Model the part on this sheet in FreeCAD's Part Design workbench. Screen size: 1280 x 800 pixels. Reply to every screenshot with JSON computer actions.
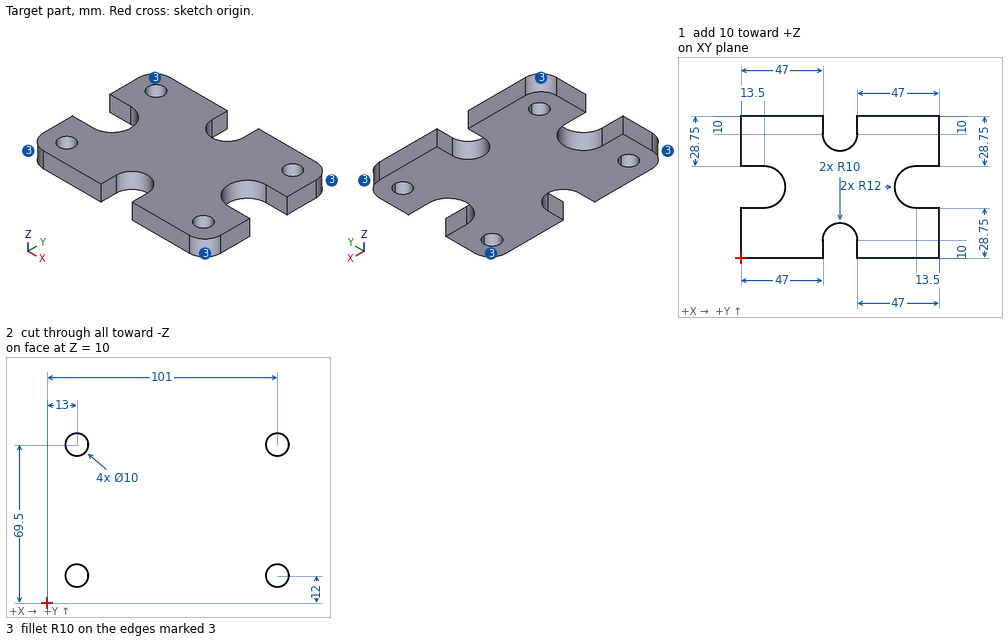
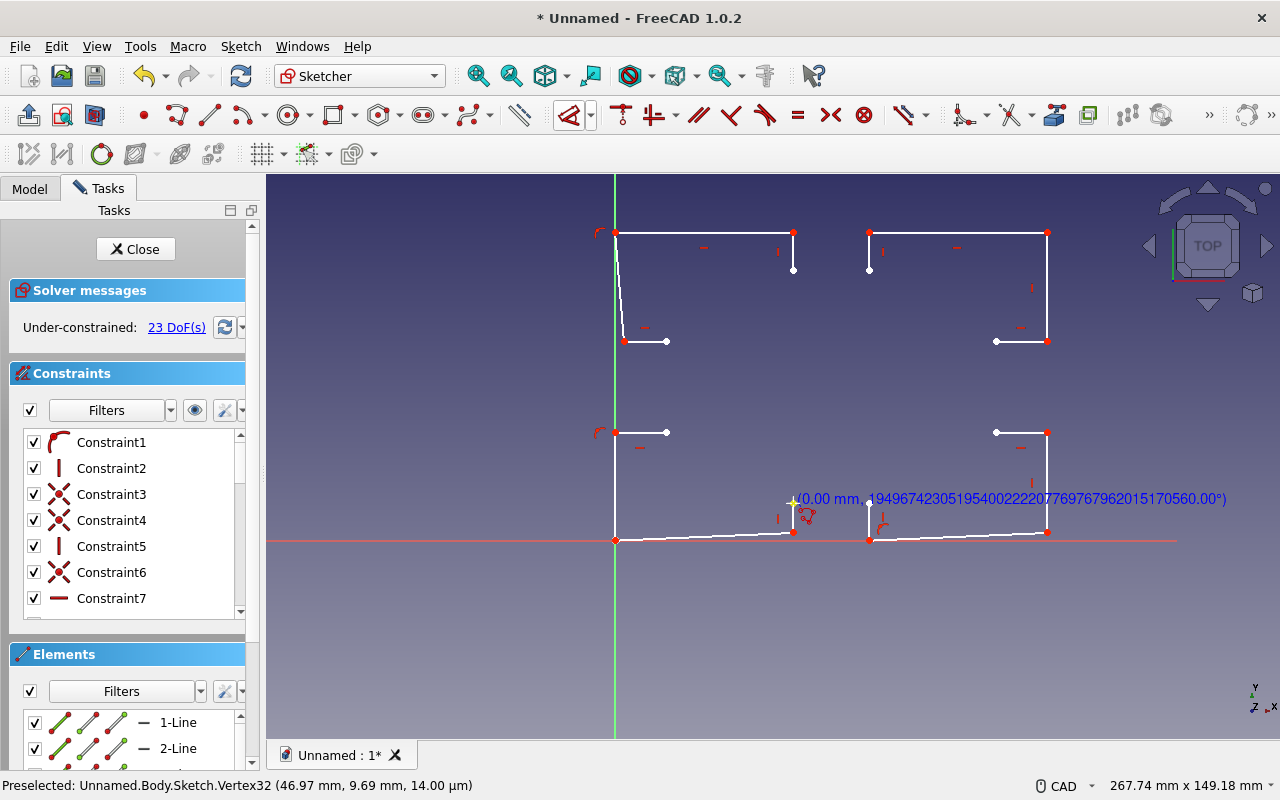
{"action": "left_click", "coordinate": [264, 116]}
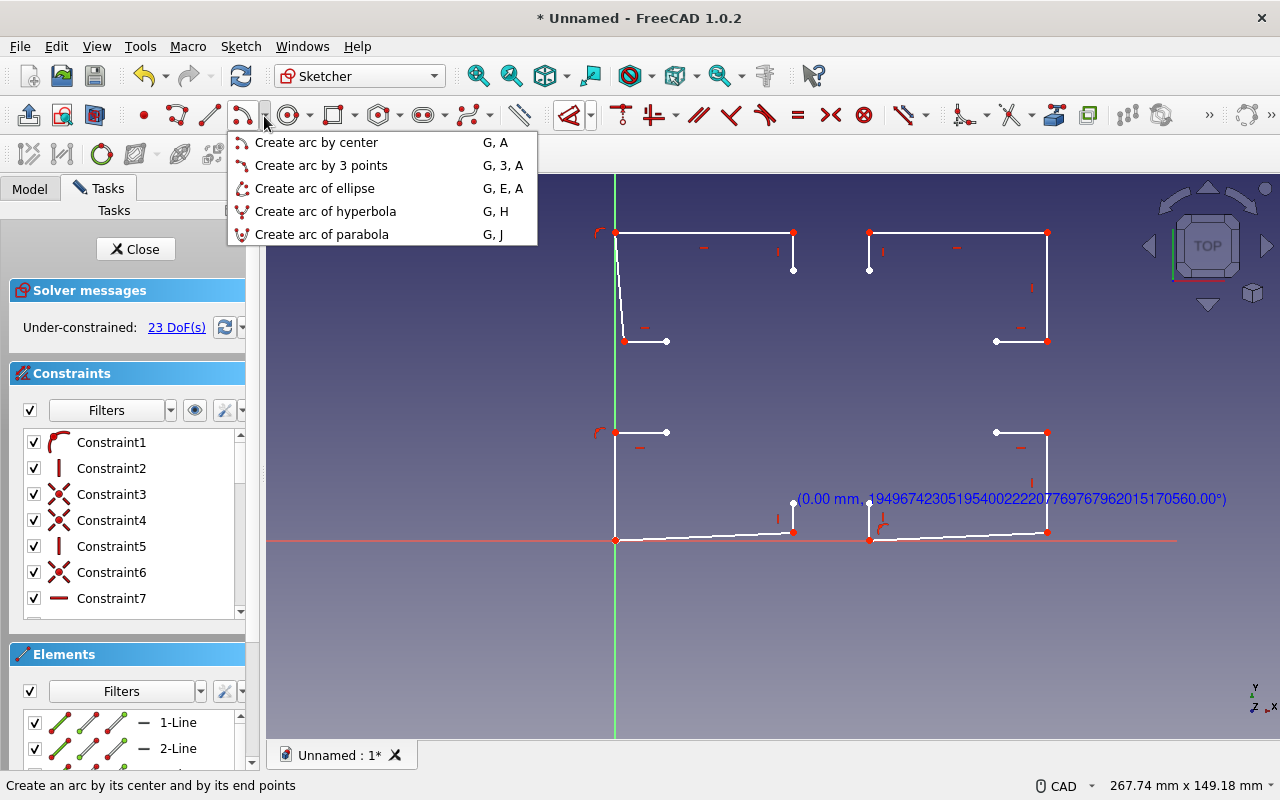
{"action": "left_click", "coordinate": [382, 166]}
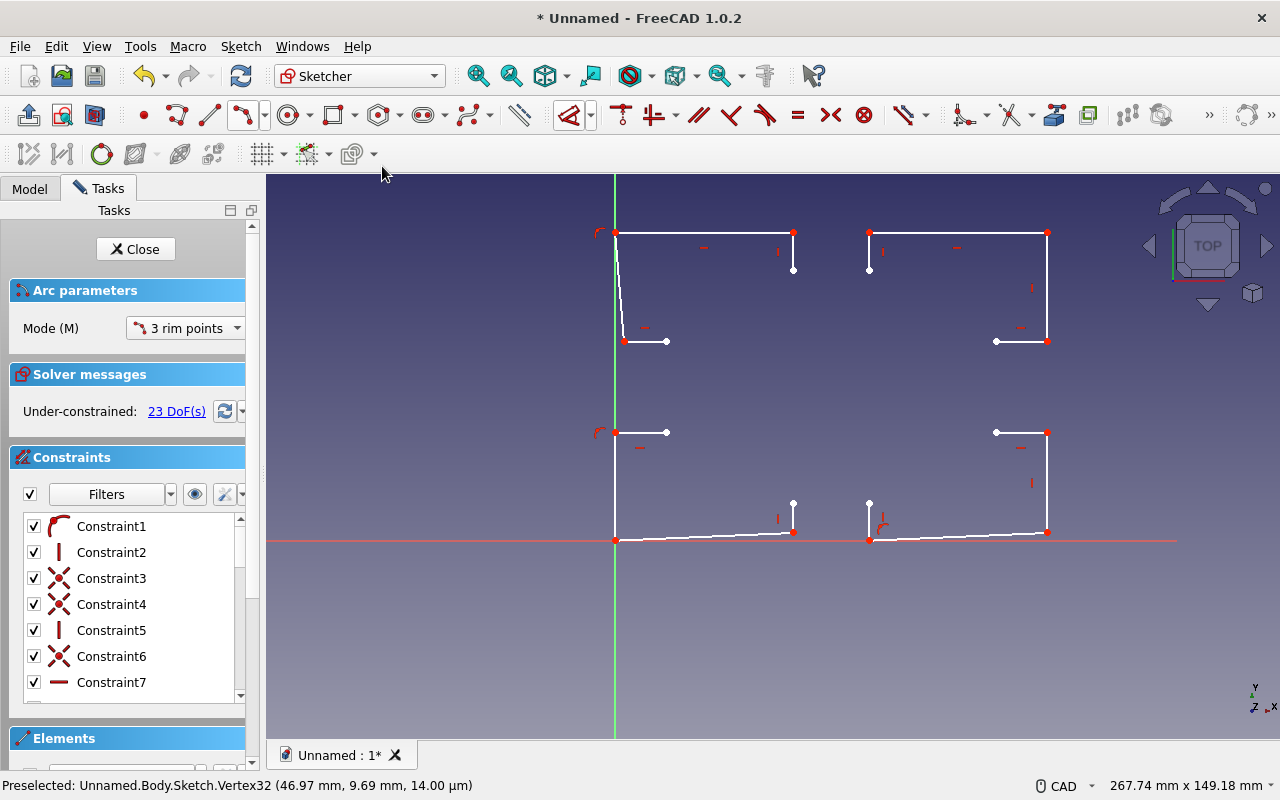
{"action": "left_click", "coordinate": [996, 433]}
{"action": "left_click", "coordinate": [996, 342]}
{"action": "left_click", "coordinate": [950, 386]}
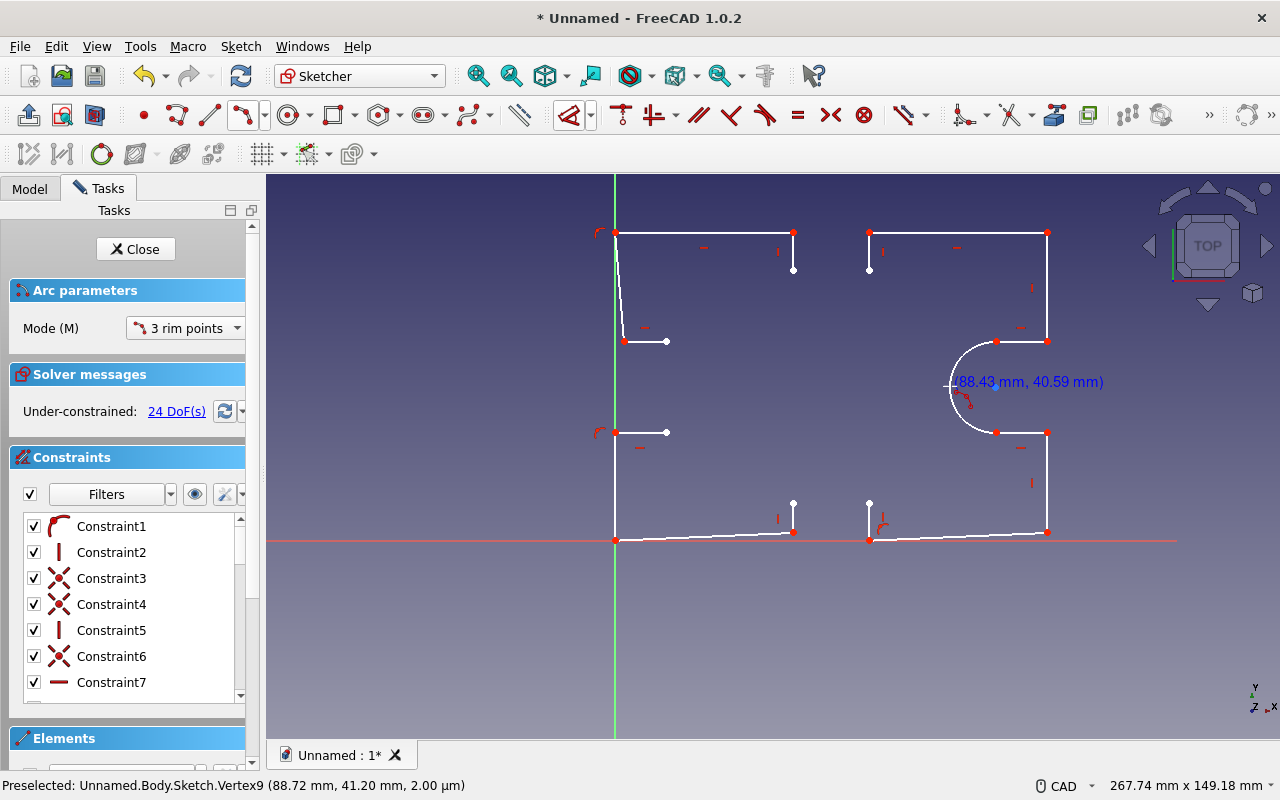
{"action": "left_click", "coordinate": [869, 271]}
{"action": "left_click", "coordinate": [793, 271]}
{"action": "left_click", "coordinate": [831, 308]}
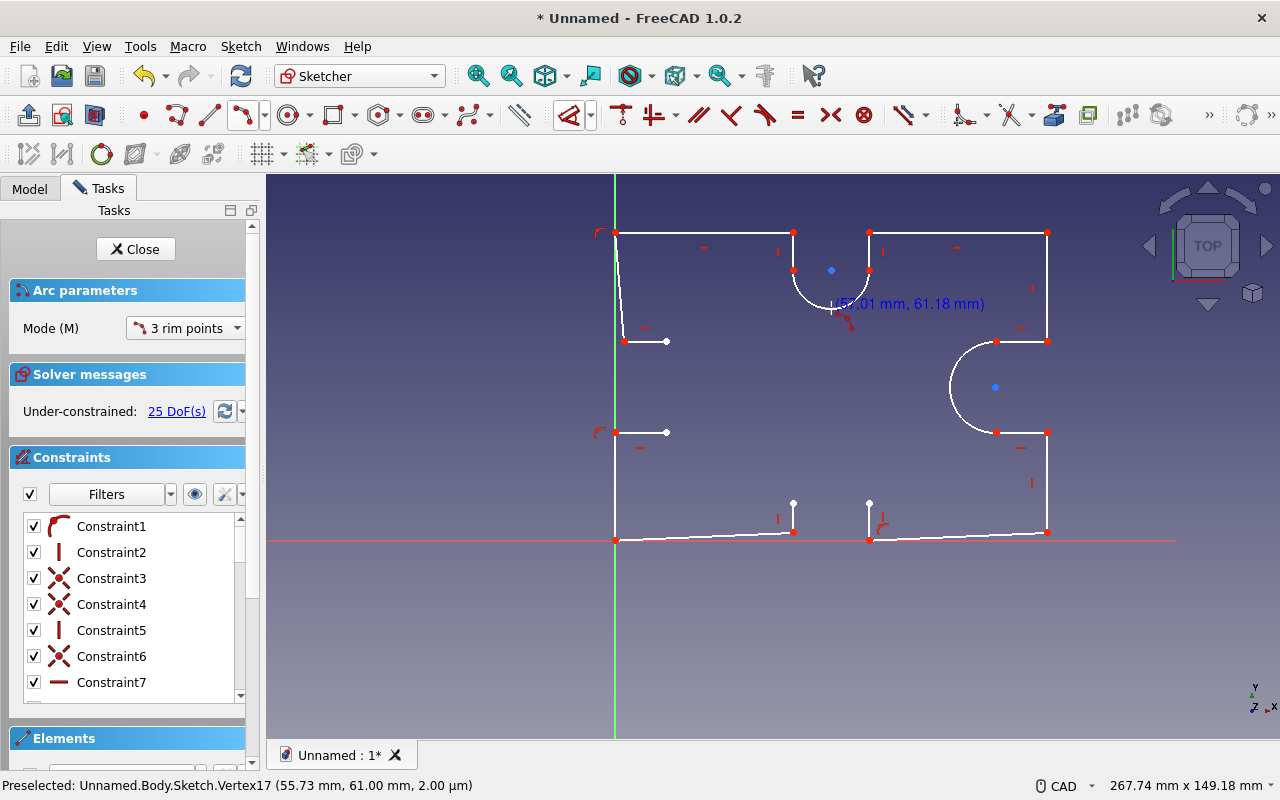
{"action": "left_click", "coordinate": [666, 342]}
{"action": "left_click", "coordinate": [666, 433]}
{"action": "left_click", "coordinate": [712, 386]}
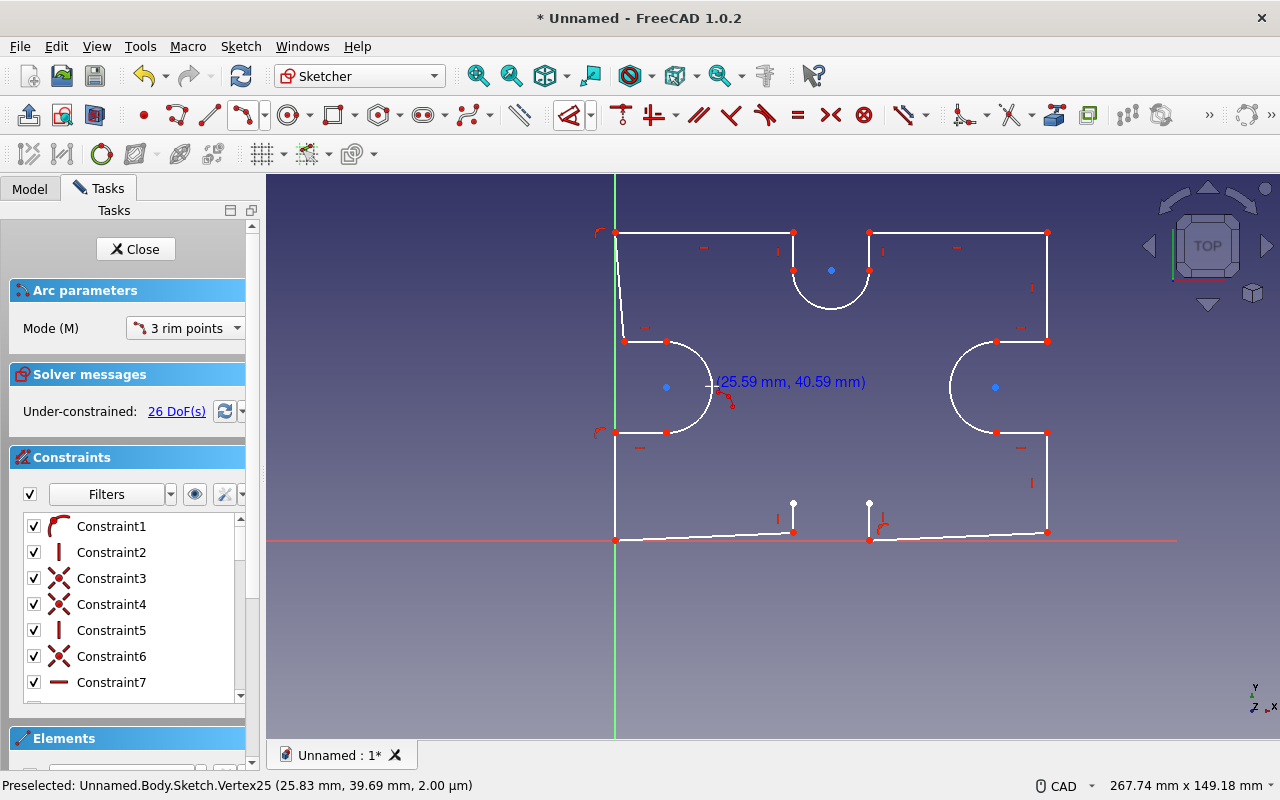
{"action": "left_click", "coordinate": [793, 504]}
{"action": "left_click", "coordinate": [869, 504]}
{"action": "left_click", "coordinate": [831, 465]}
{"action": "key", "text": "Escape"}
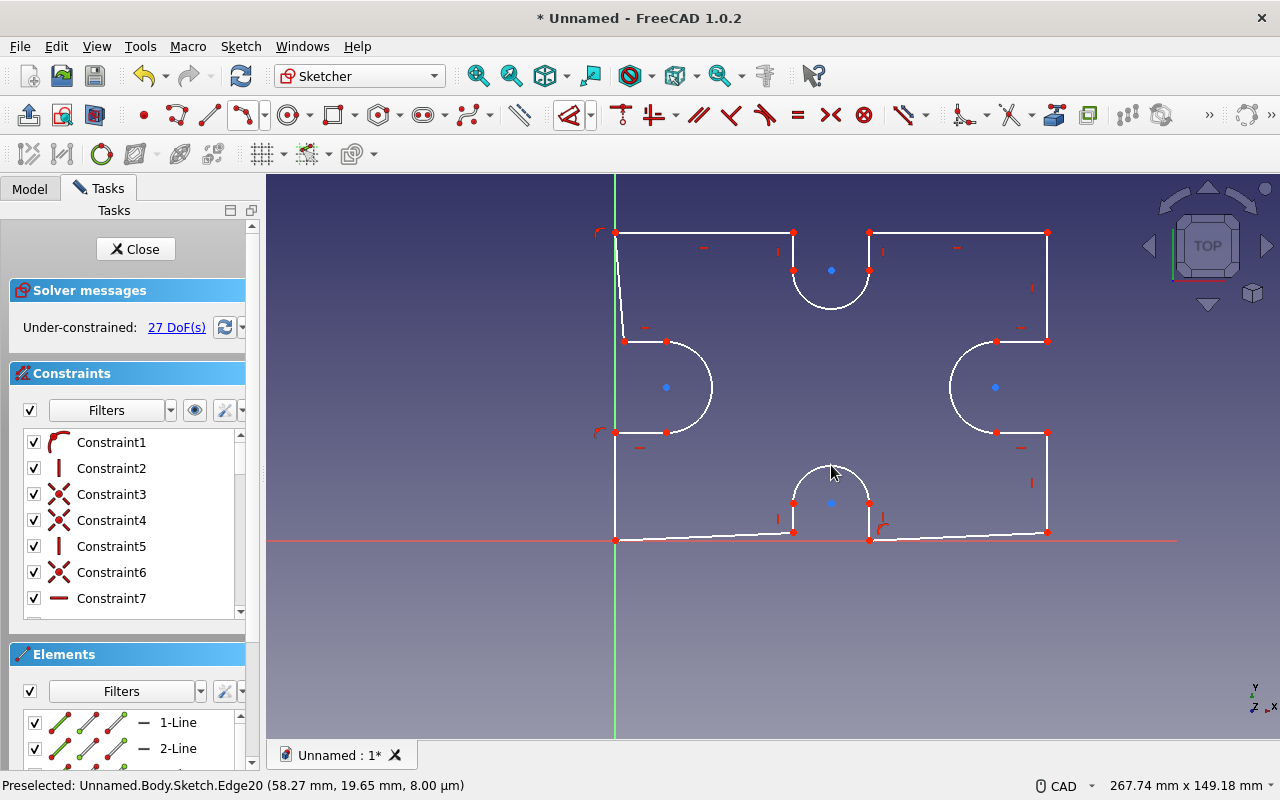
{"action": "scroll", "coordinate": [869, 515], "scroll_direction": "up", "scroll_amount": 2}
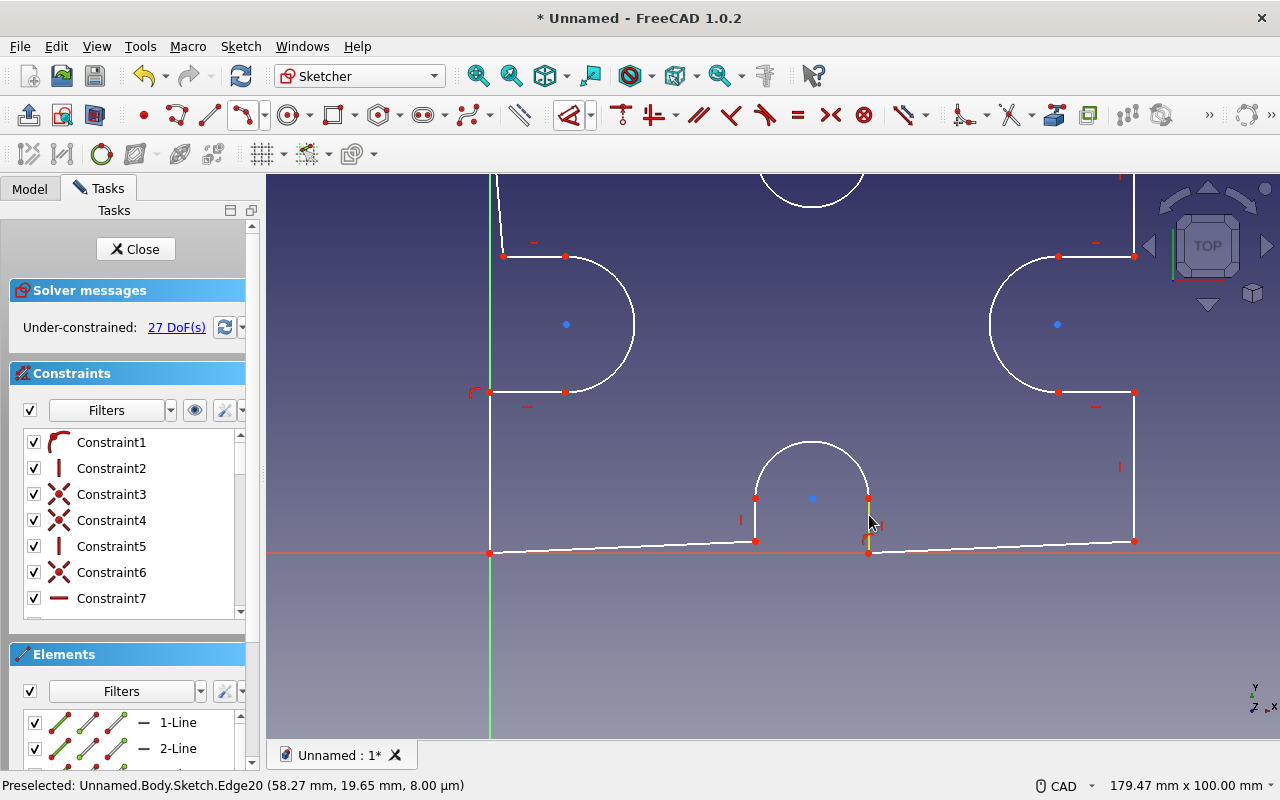
{"action": "left_click", "coordinate": [869, 515]}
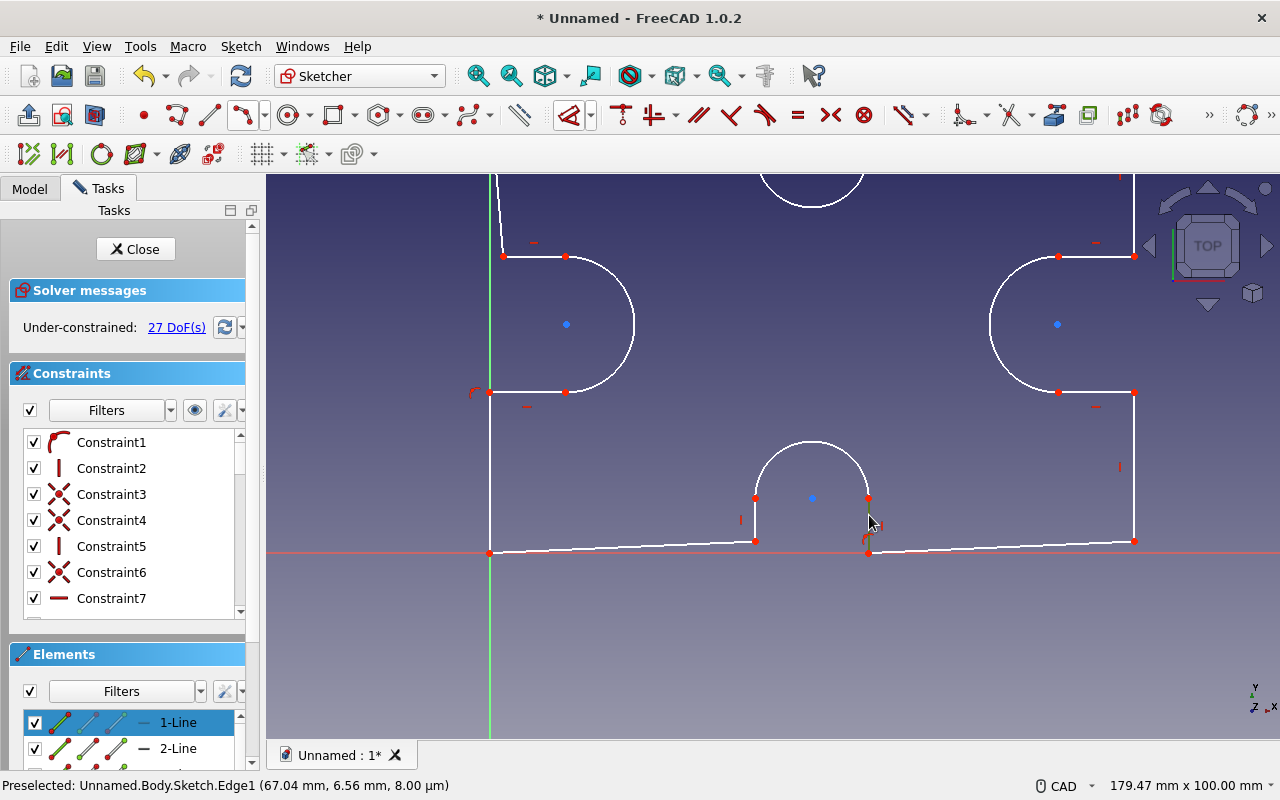
{"action": "left_click", "coordinate": [845, 452]}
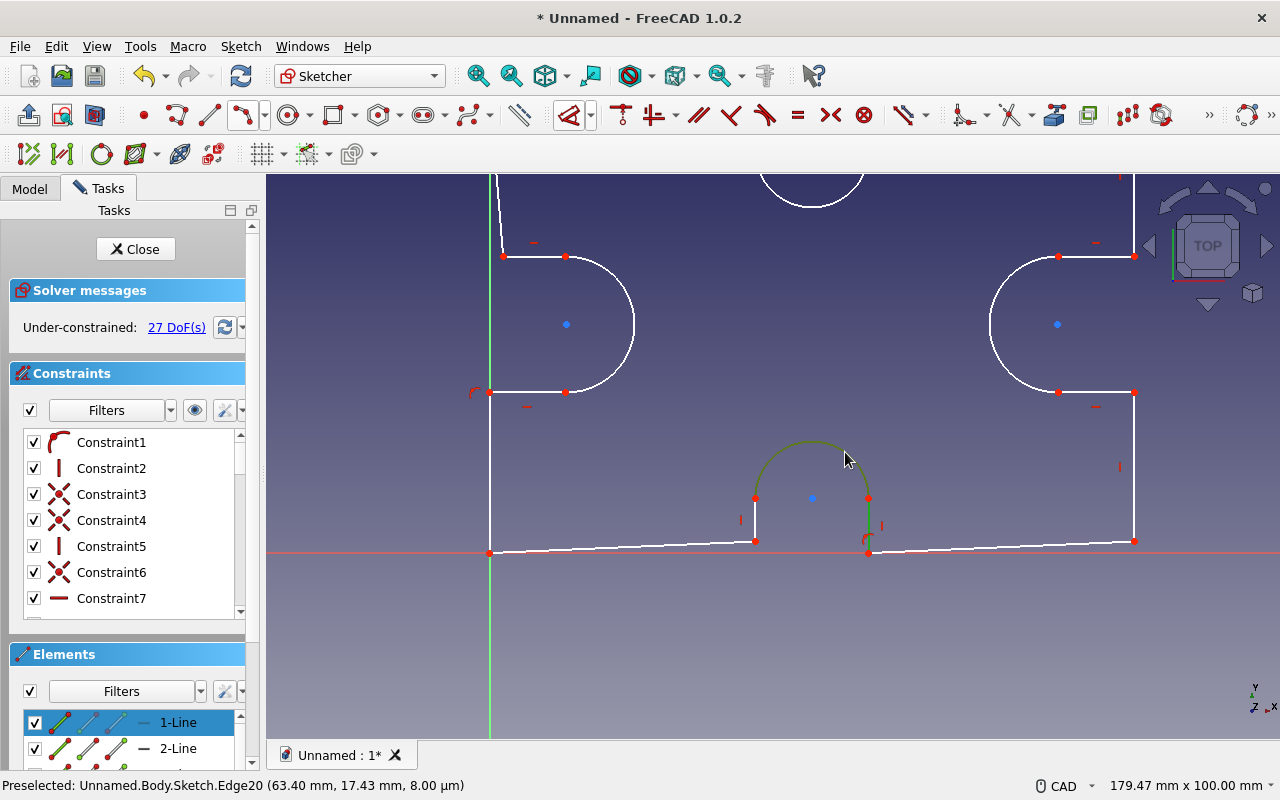
{"action": "left_click", "coordinate": [765, 116]}